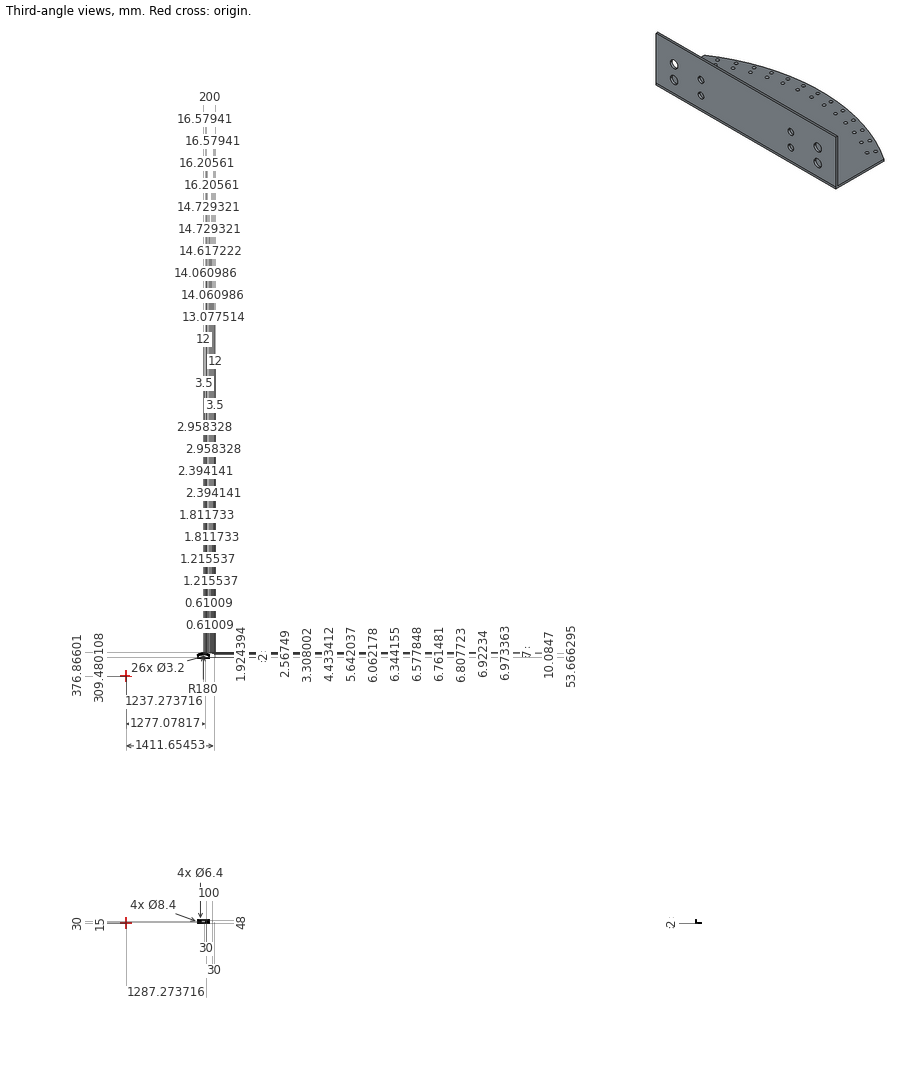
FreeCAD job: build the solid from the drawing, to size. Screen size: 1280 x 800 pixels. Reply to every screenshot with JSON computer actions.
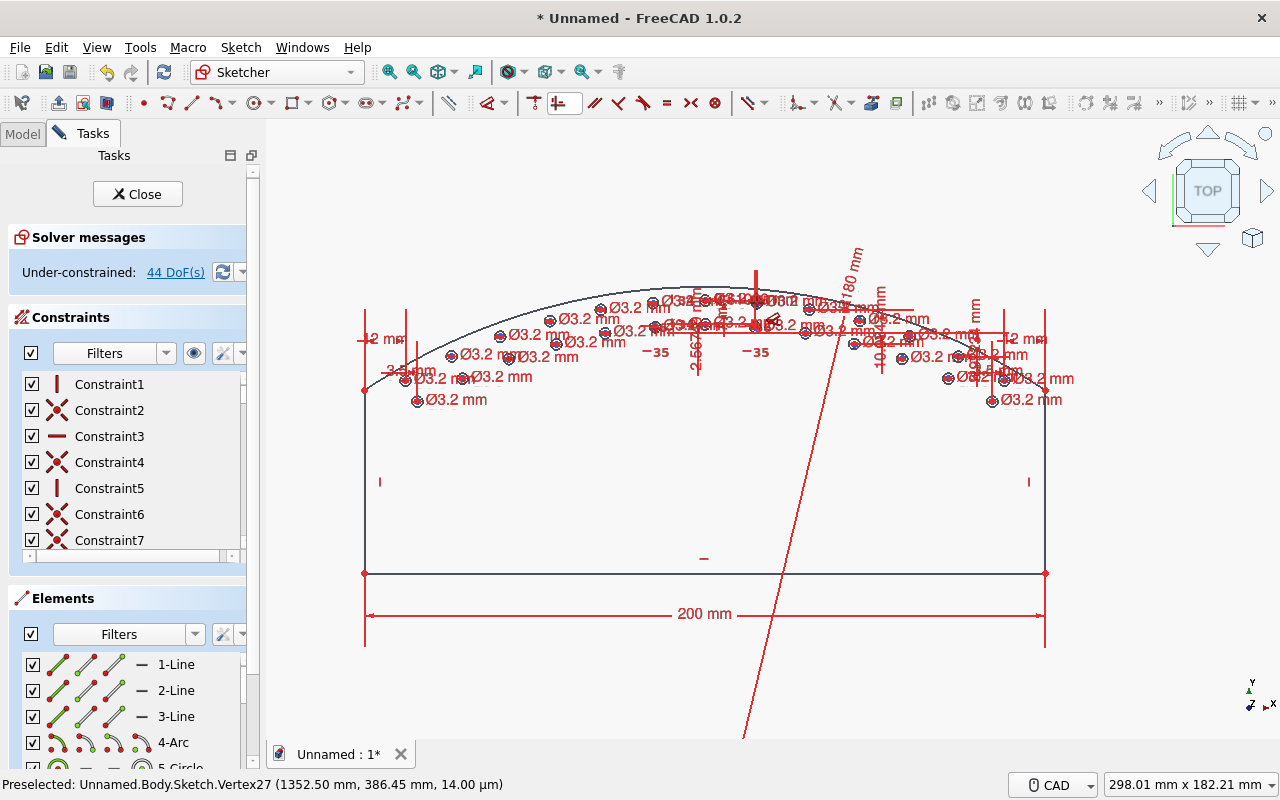
{"action": "scroll", "coordinate": [705, 324], "scroll_direction": "up", "scroll_amount": 8}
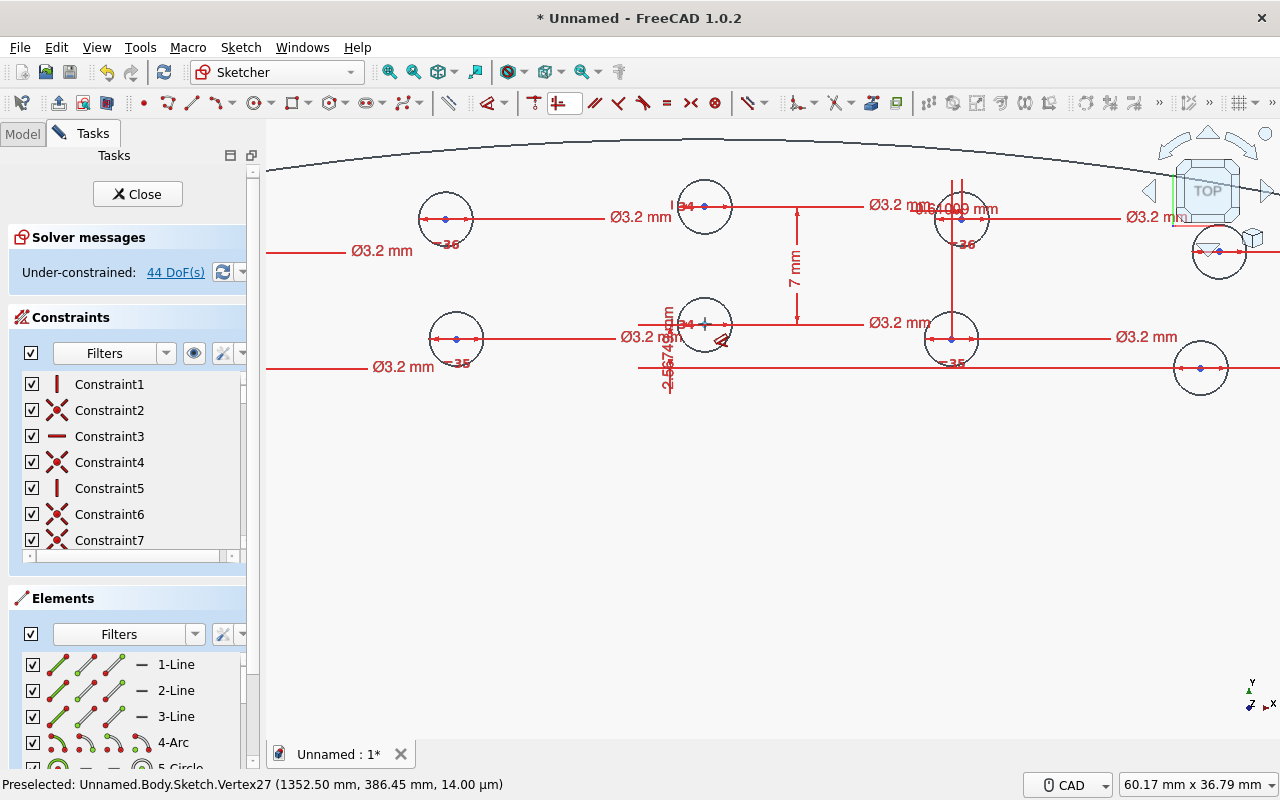
{"action": "left_click", "coordinate": [705, 325]}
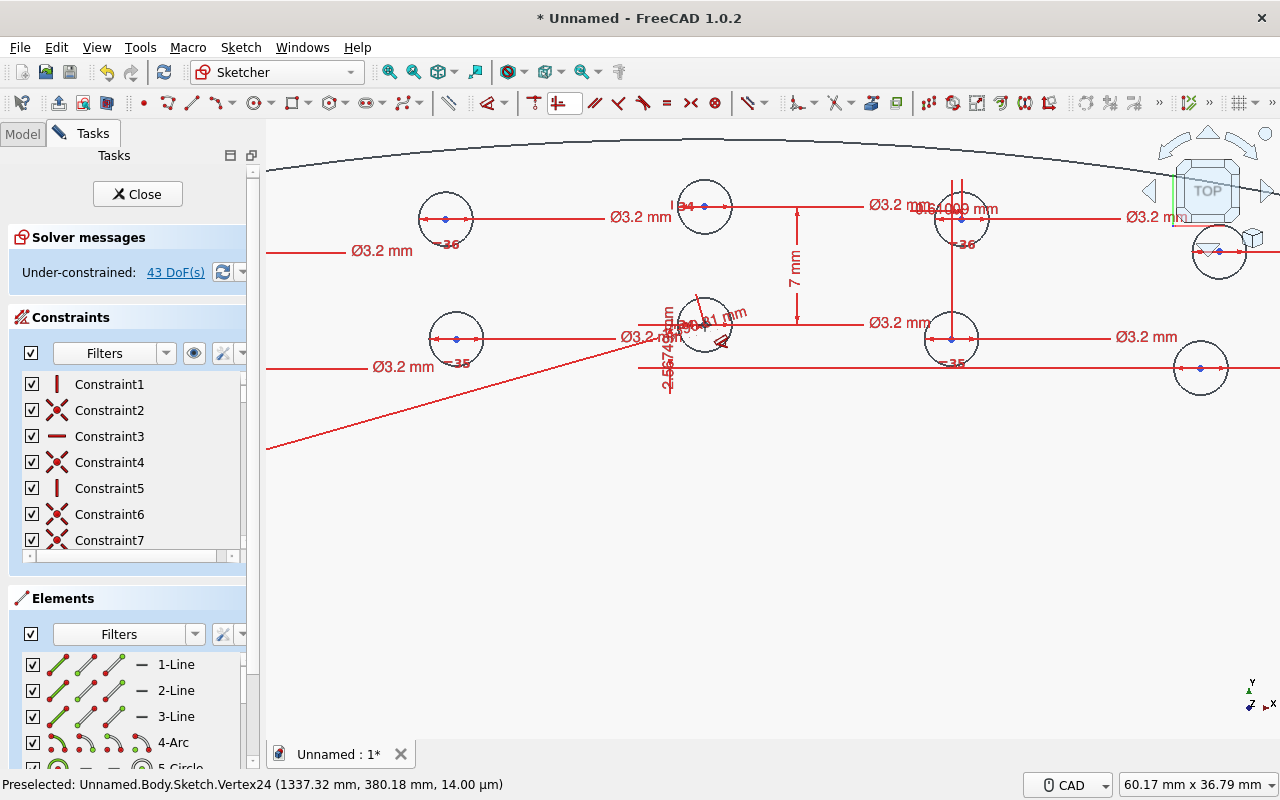
{"action": "scroll", "coordinate": [705, 347], "scroll_direction": "down", "scroll_amount": 9}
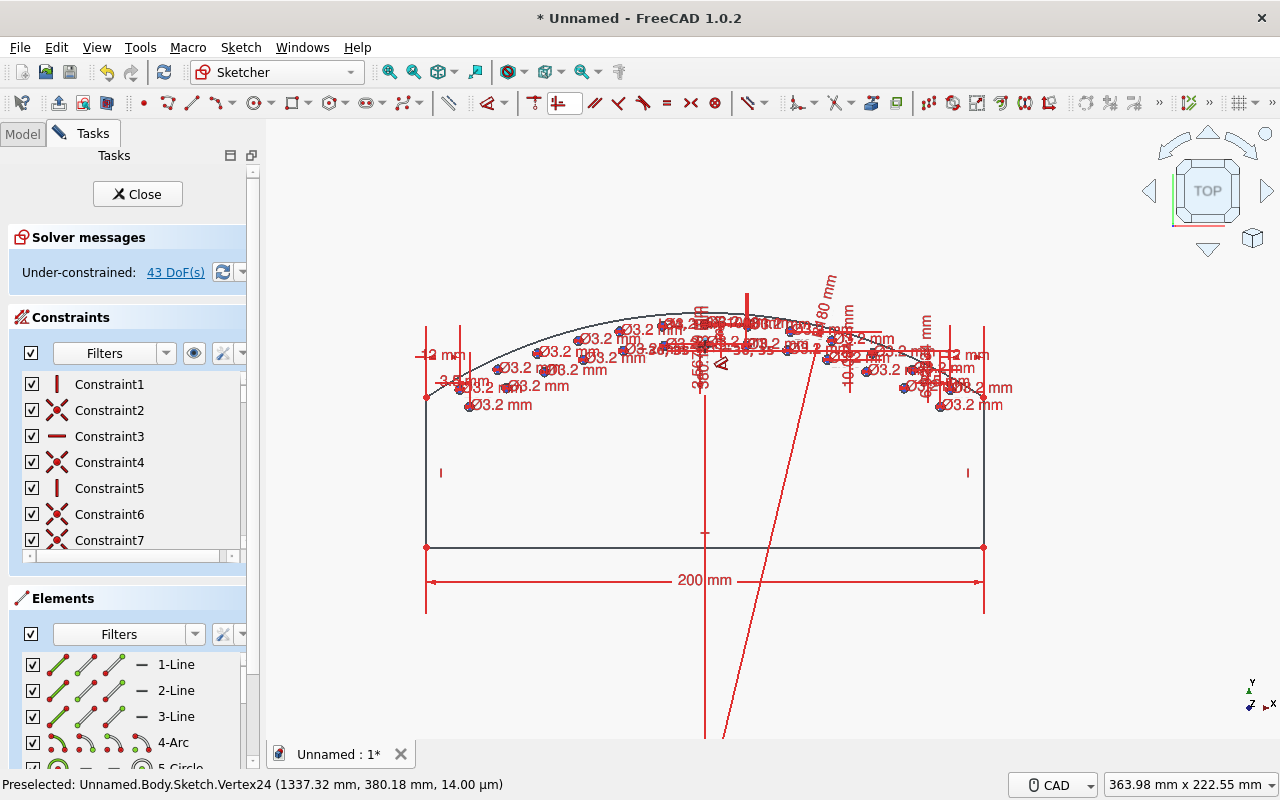
{"action": "scroll", "coordinate": [623, 351], "scroll_direction": "up", "scroll_amount": 9}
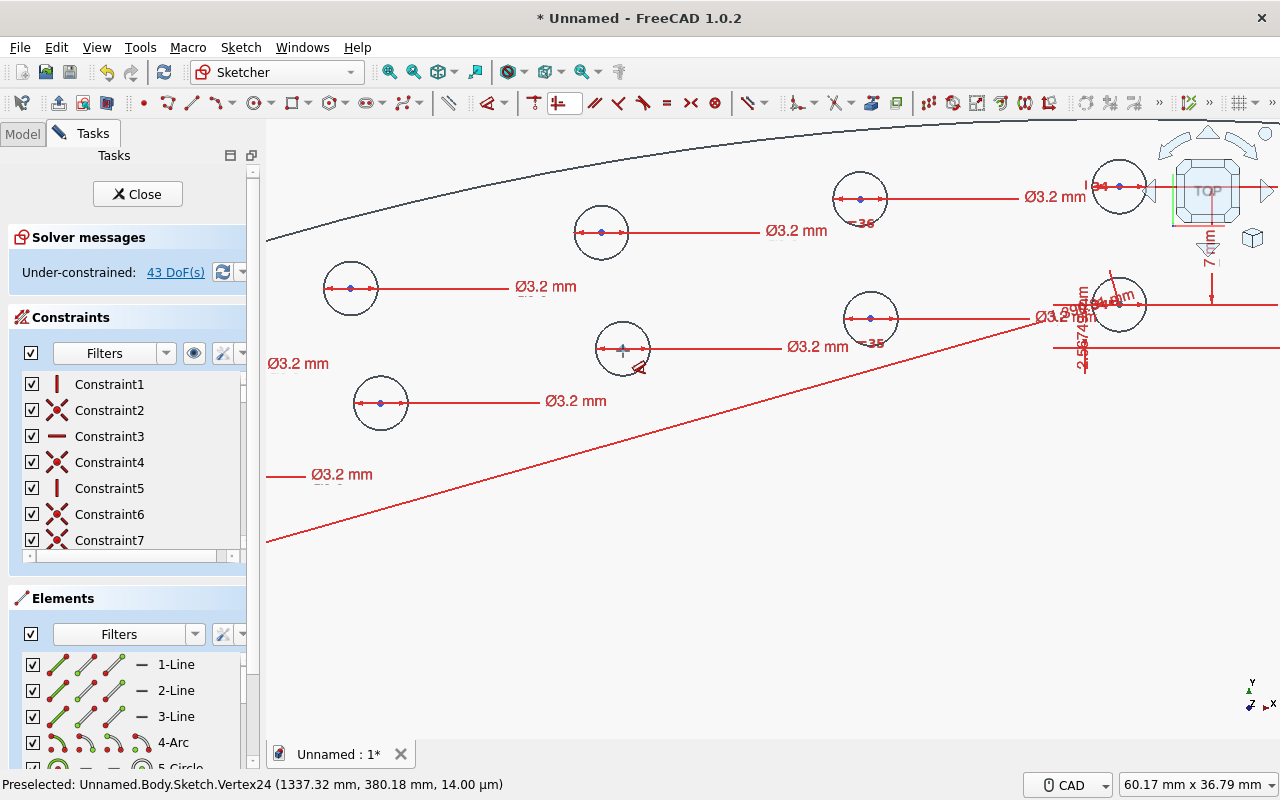
{"action": "left_click", "coordinate": [623, 349]}
{"action": "left_click", "coordinate": [589, 327]}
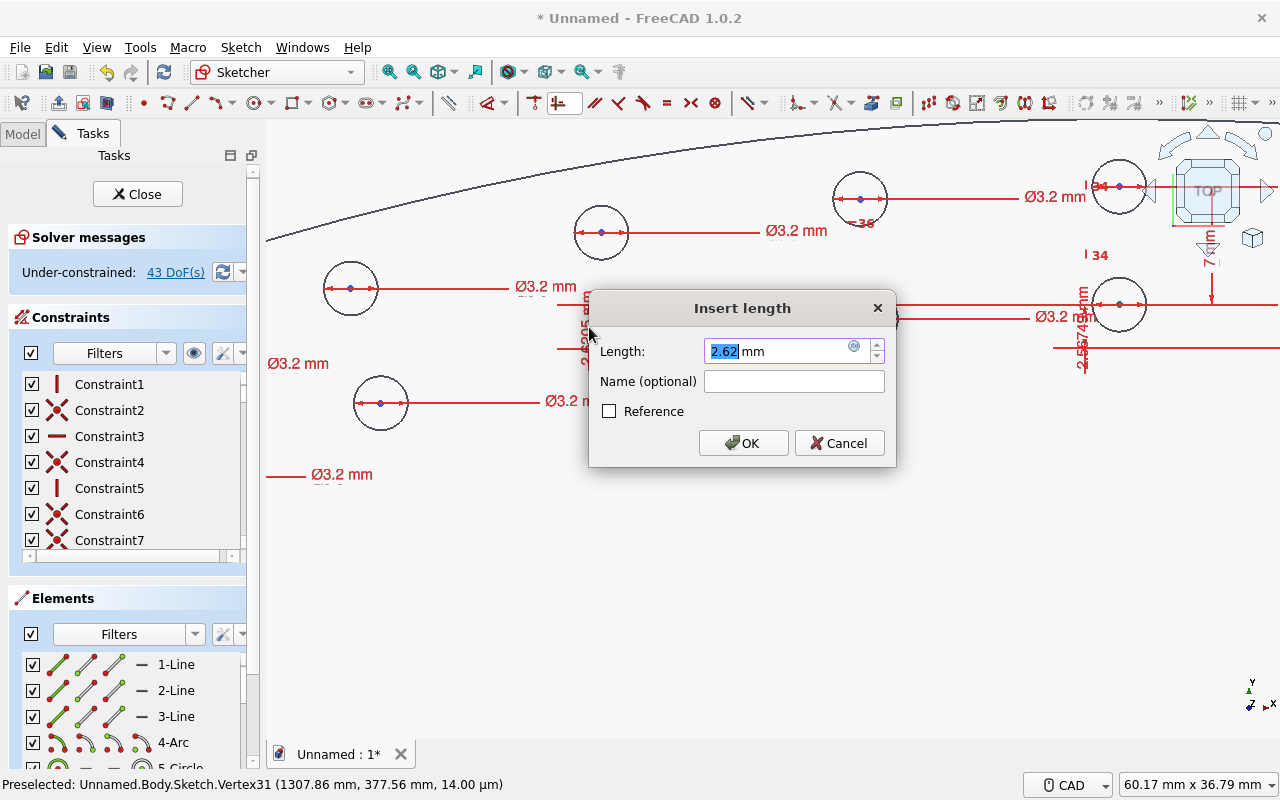
{"action": "type", "text": "2.56749"}
{"action": "key", "text": "Return"}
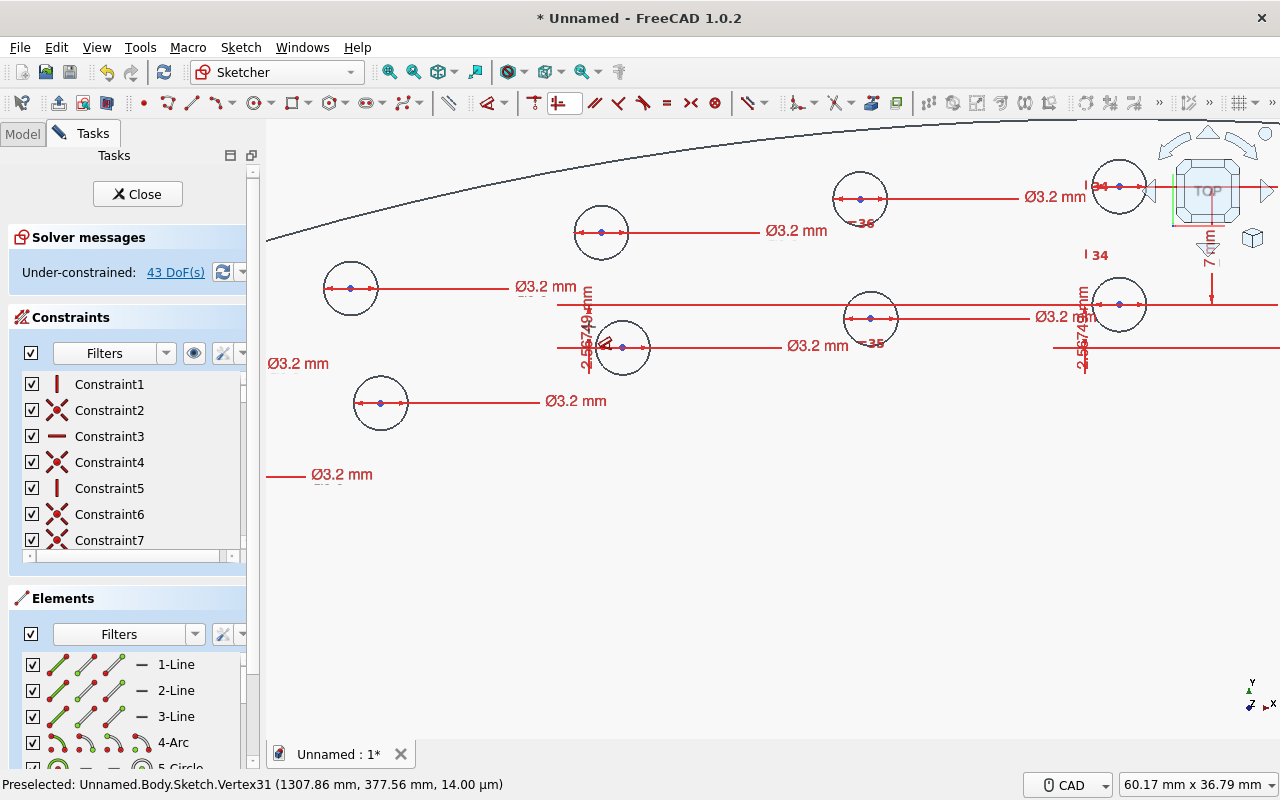
{"action": "scroll", "coordinate": [623, 351], "scroll_direction": "down", "scroll_amount": 9}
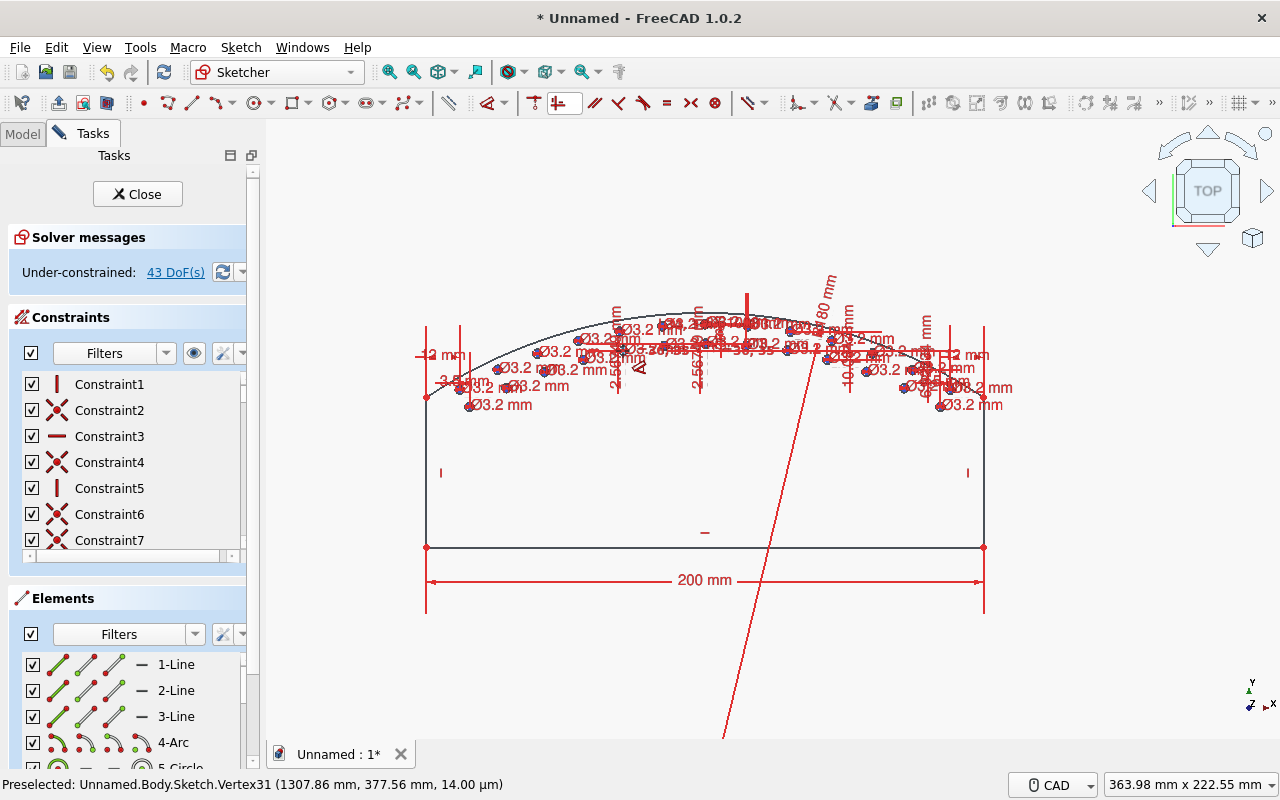
{"action": "scroll", "coordinate": [583, 360], "scroll_direction": "up", "scroll_amount": 2}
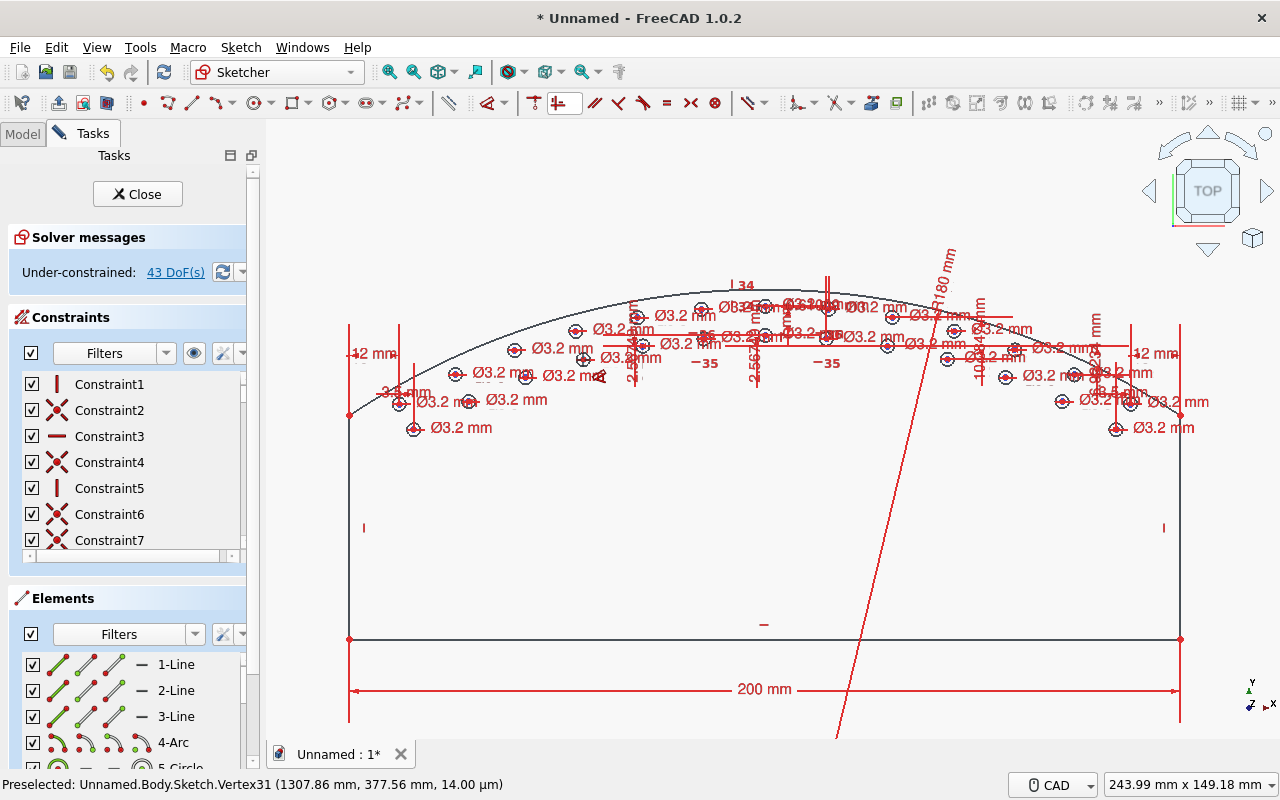
{"action": "left_click", "coordinate": [583, 360]}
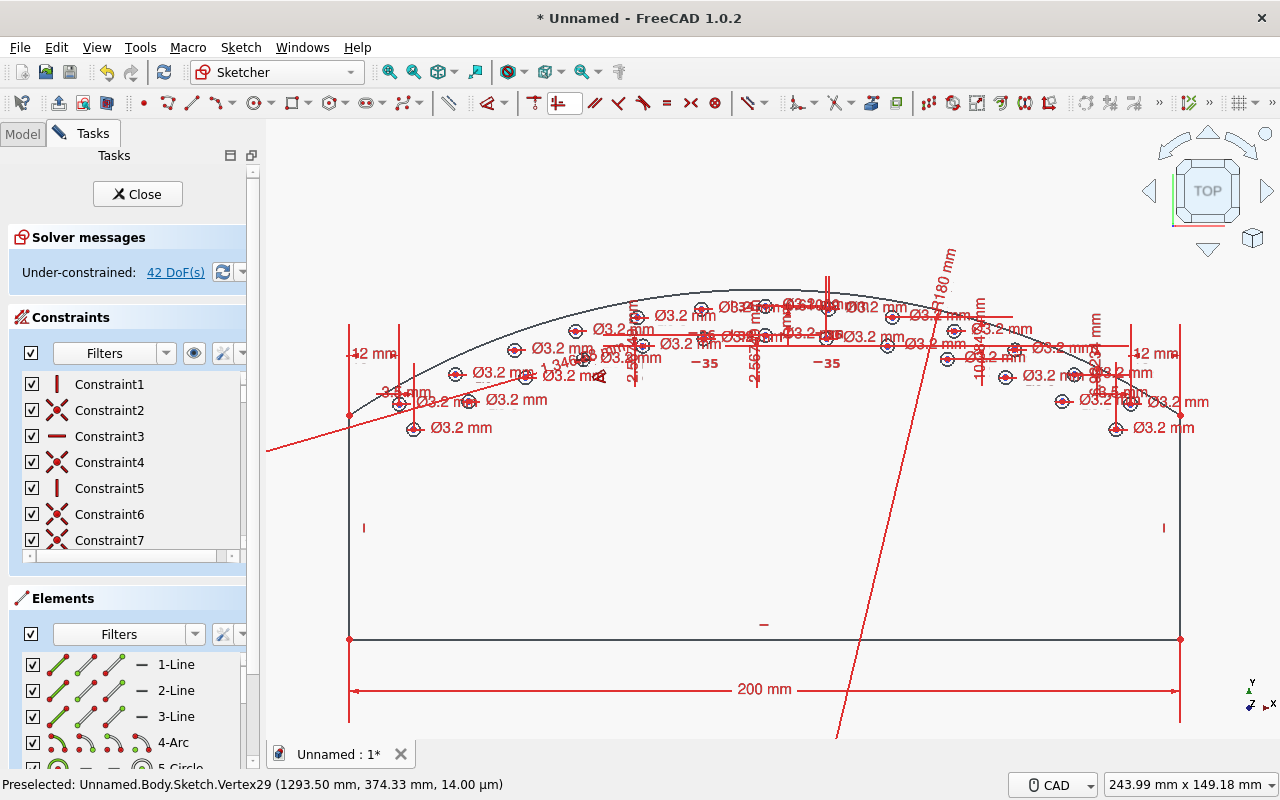
{"action": "left_click", "coordinate": [638, 318]}
{"action": "left_click", "coordinate": [549, 339]}